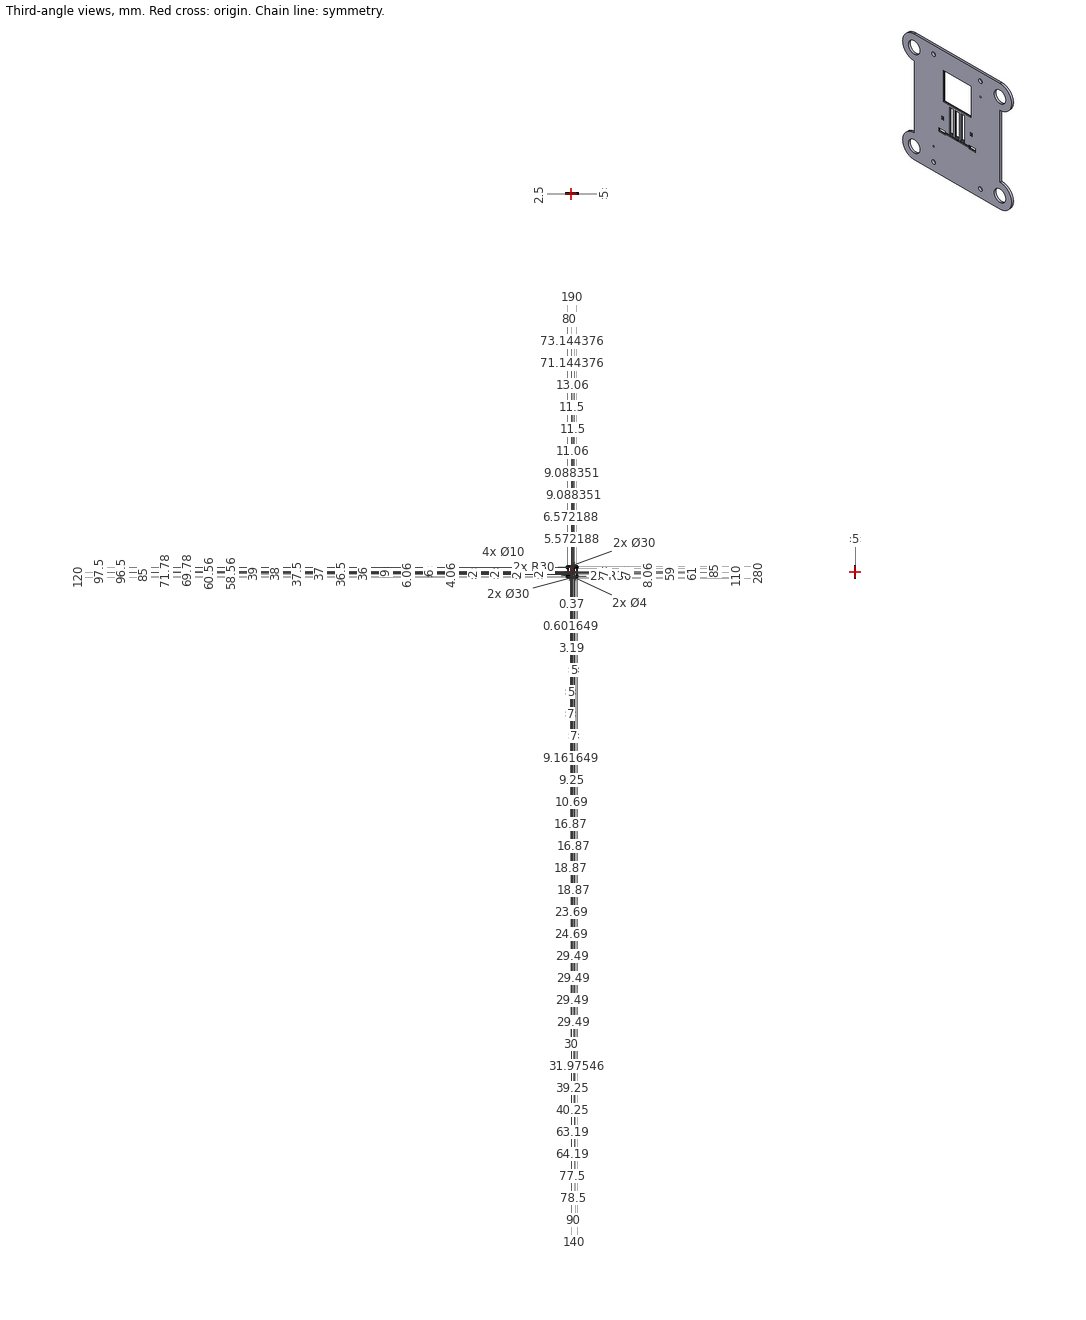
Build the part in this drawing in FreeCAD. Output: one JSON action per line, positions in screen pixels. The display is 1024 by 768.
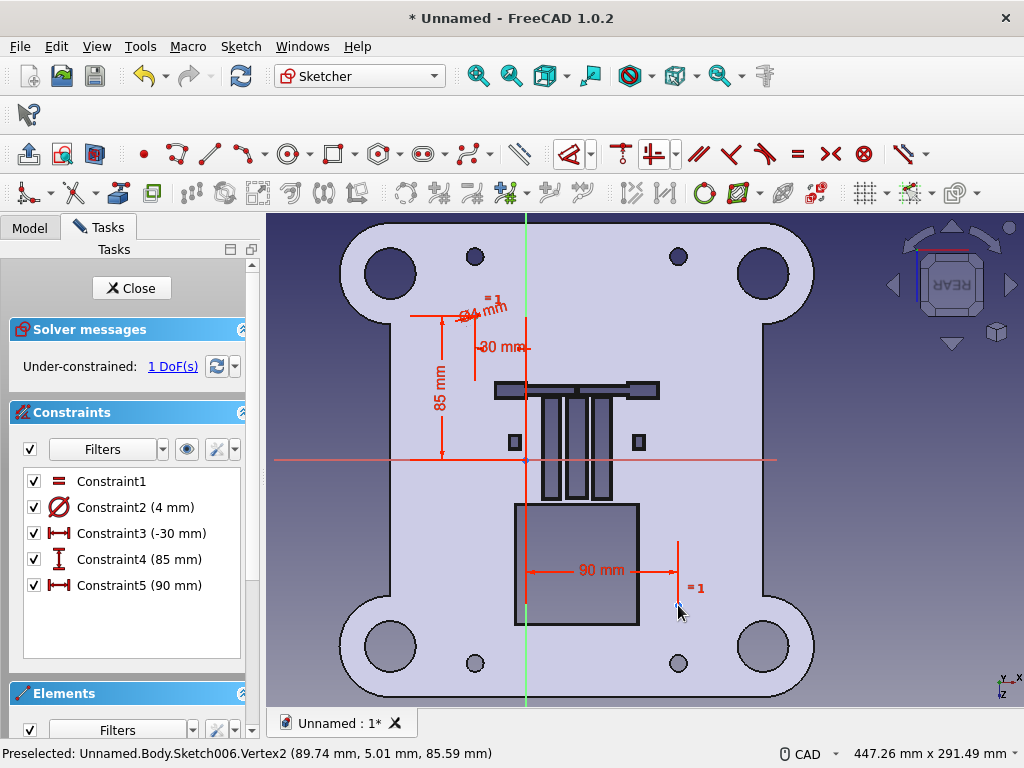
{"action": "left_click", "coordinate": [678, 605]}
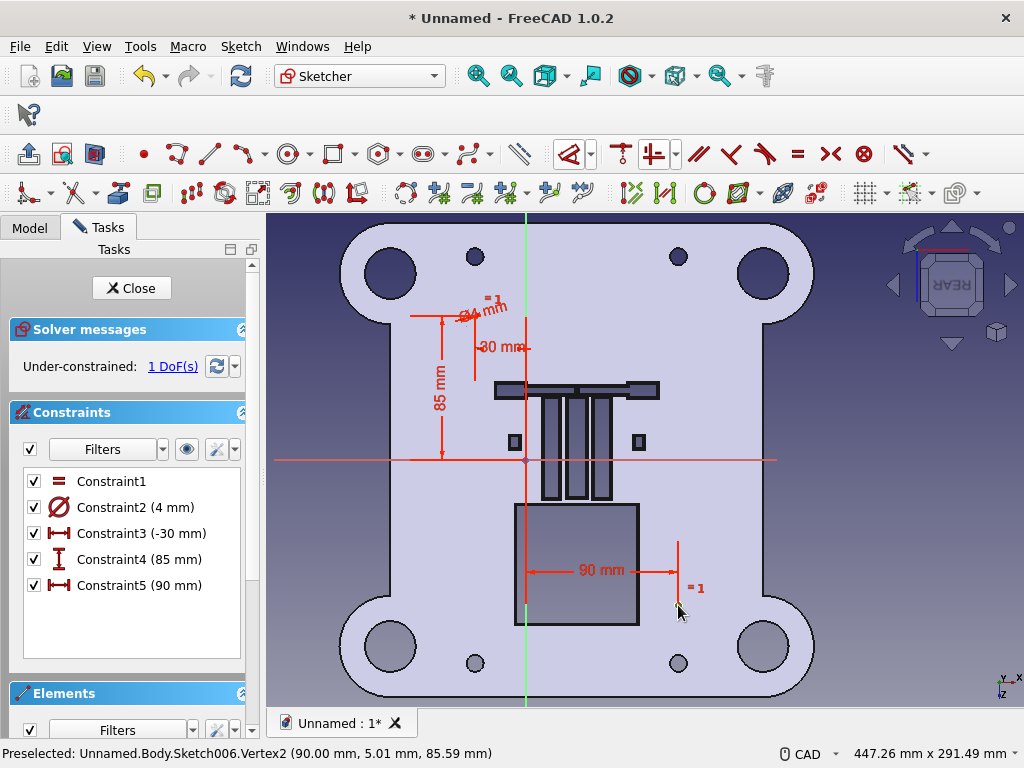
{"action": "left_click", "coordinate": [590, 154]}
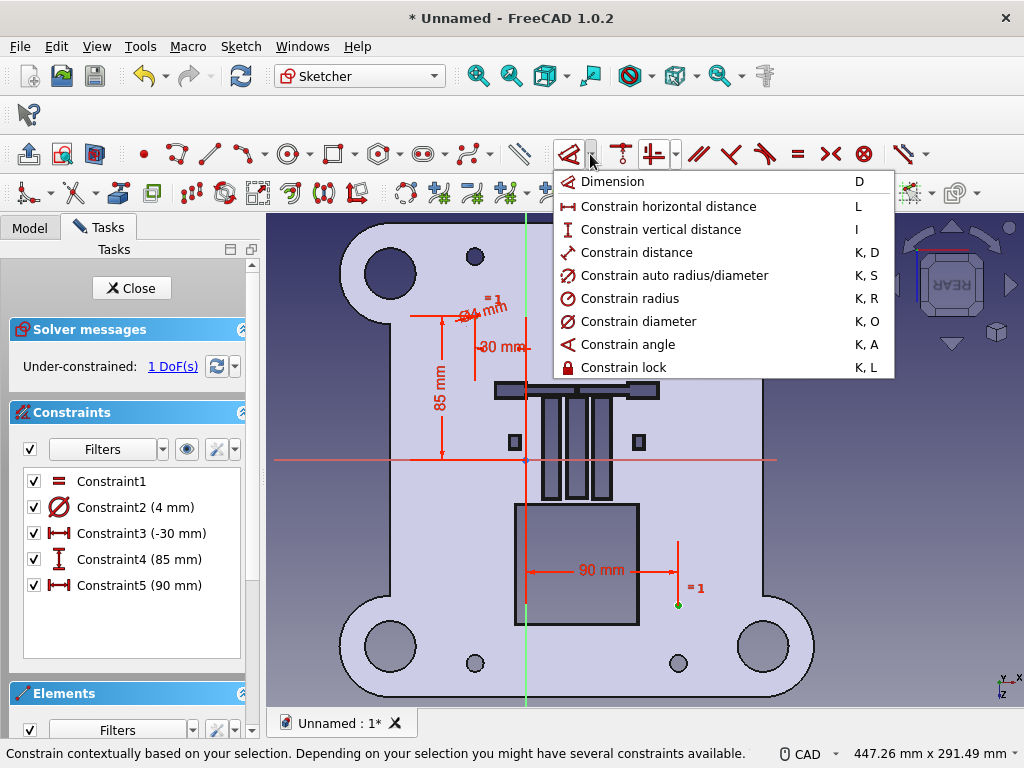
{"action": "left_click", "coordinate": [724, 230]}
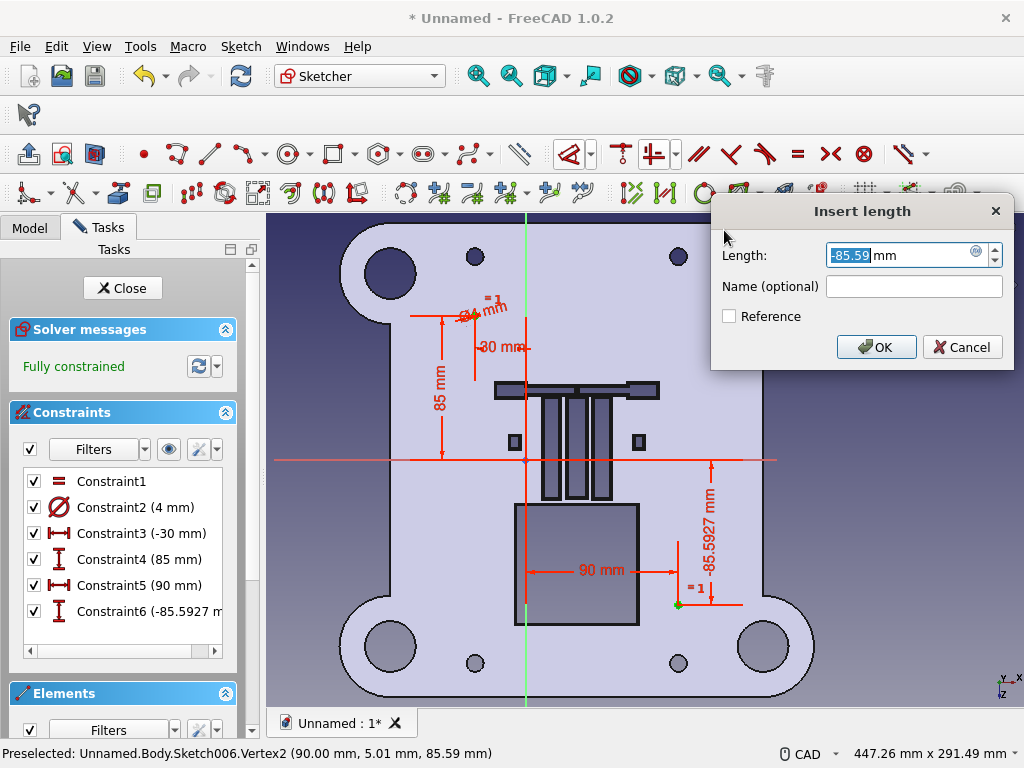
{"action": "type", "text": "-85"}
{"action": "key", "text": "Return"}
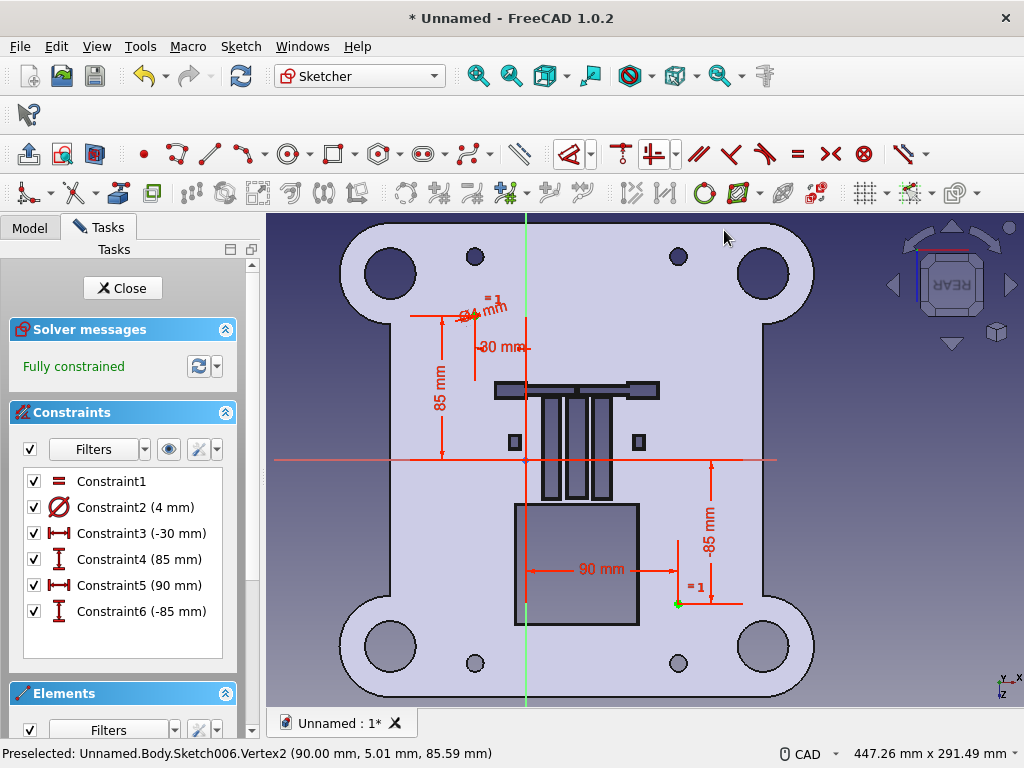
{"action": "left_click", "coordinate": [123, 288]}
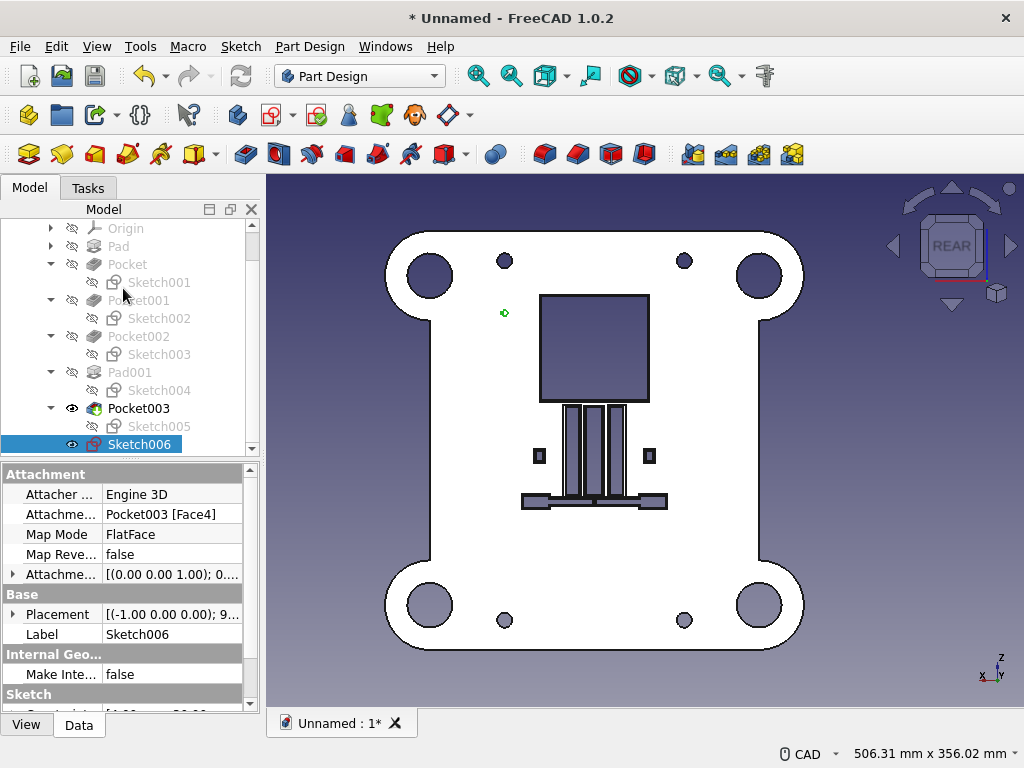
{"action": "left_click", "coordinate": [246, 154]}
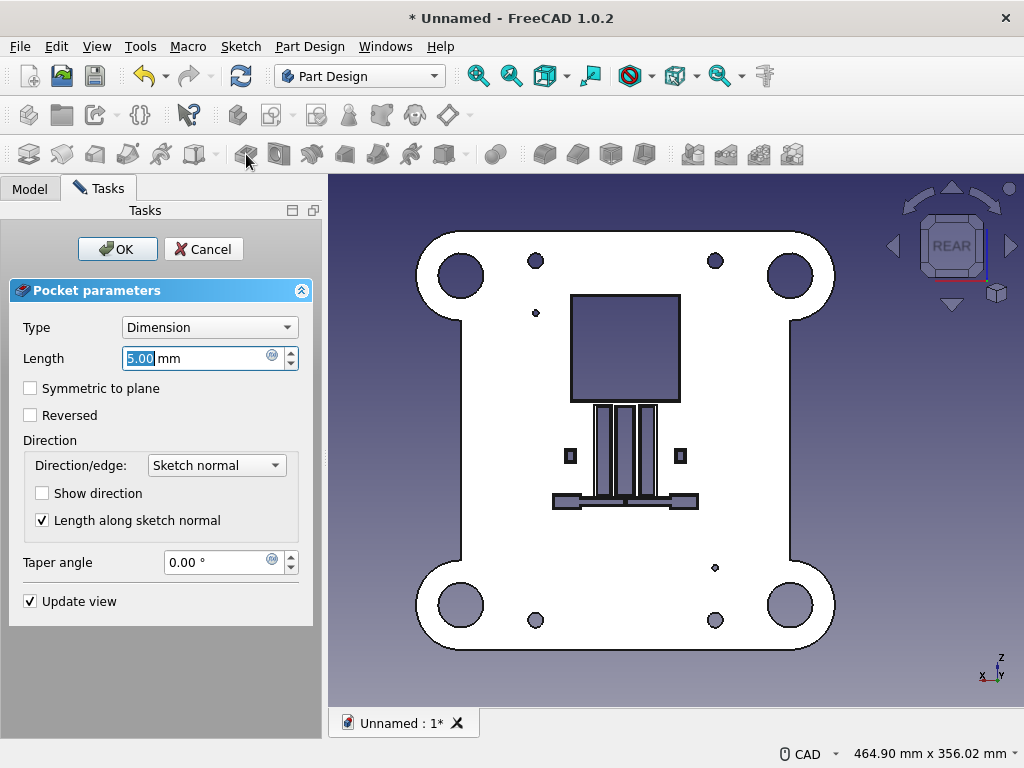
{"action": "left_click", "coordinate": [210, 328]}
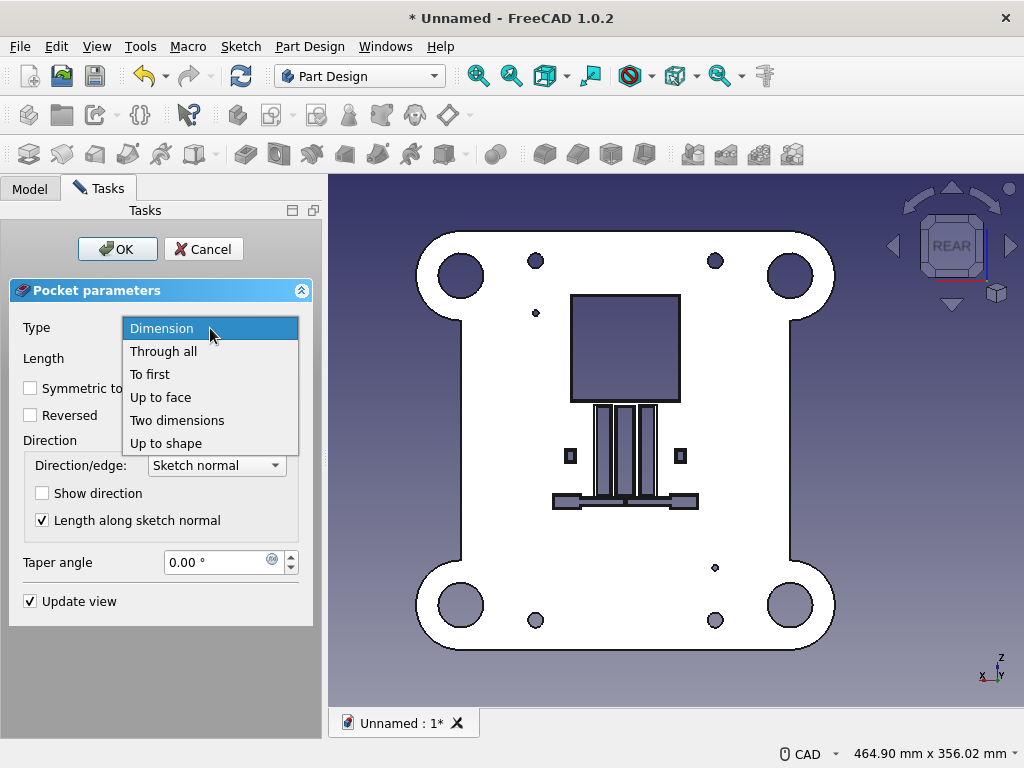
{"action": "left_click", "coordinate": [208, 352]}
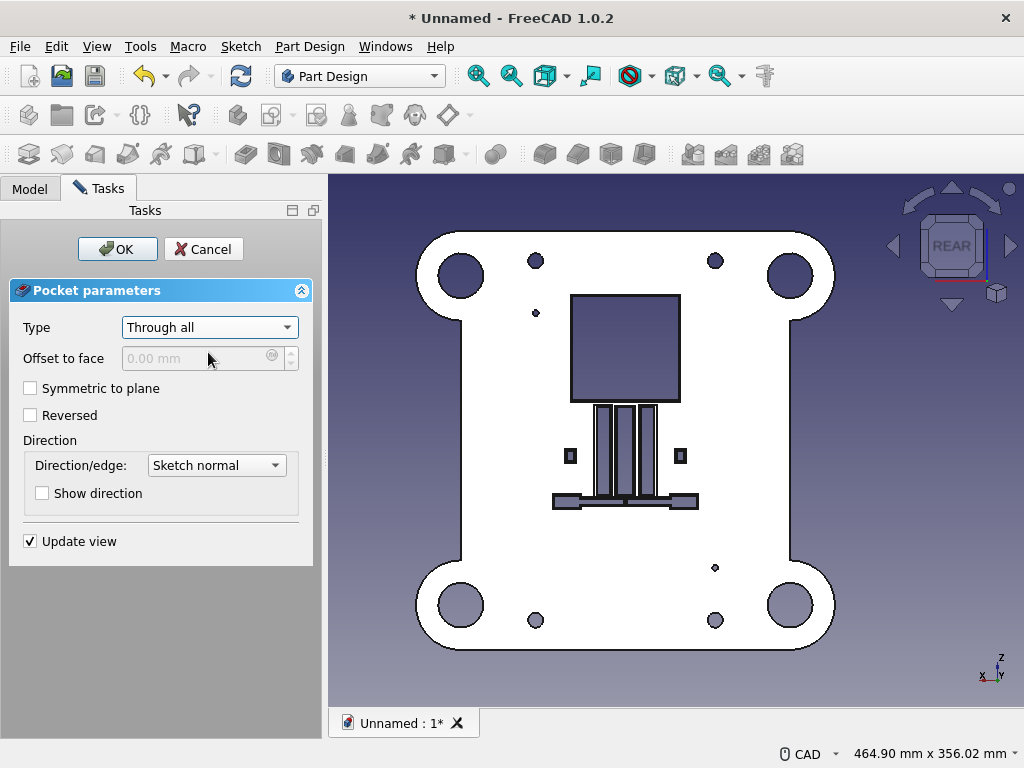
{"action": "left_click", "coordinate": [118, 249]}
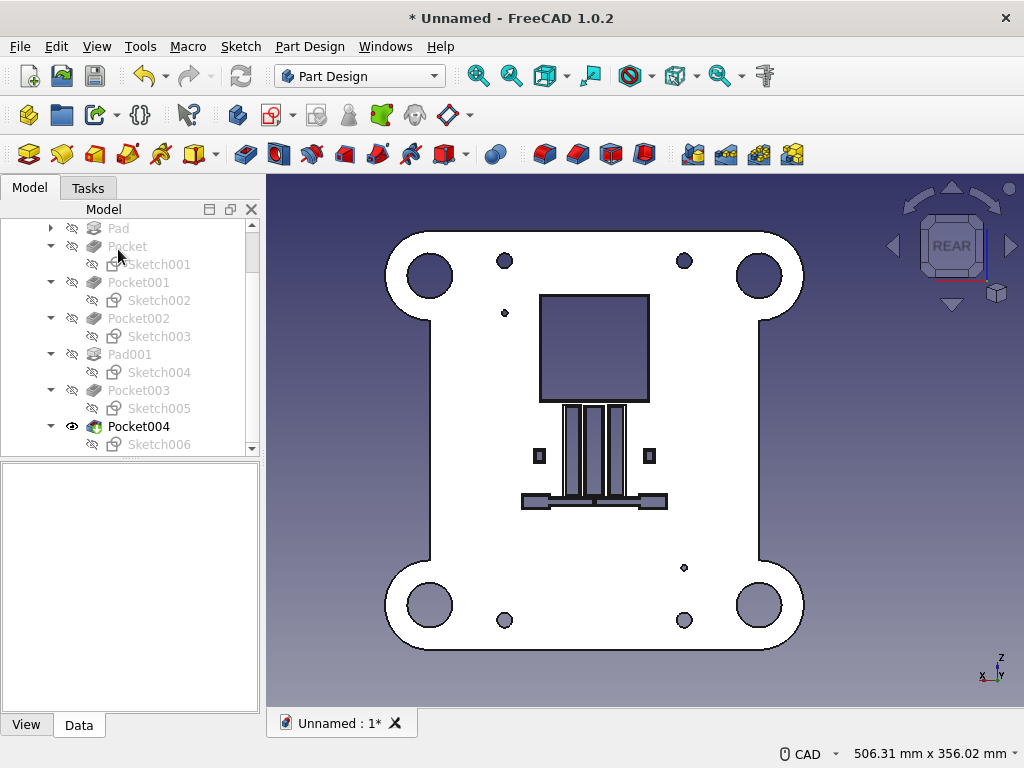
{"action": "key", "text": "0"}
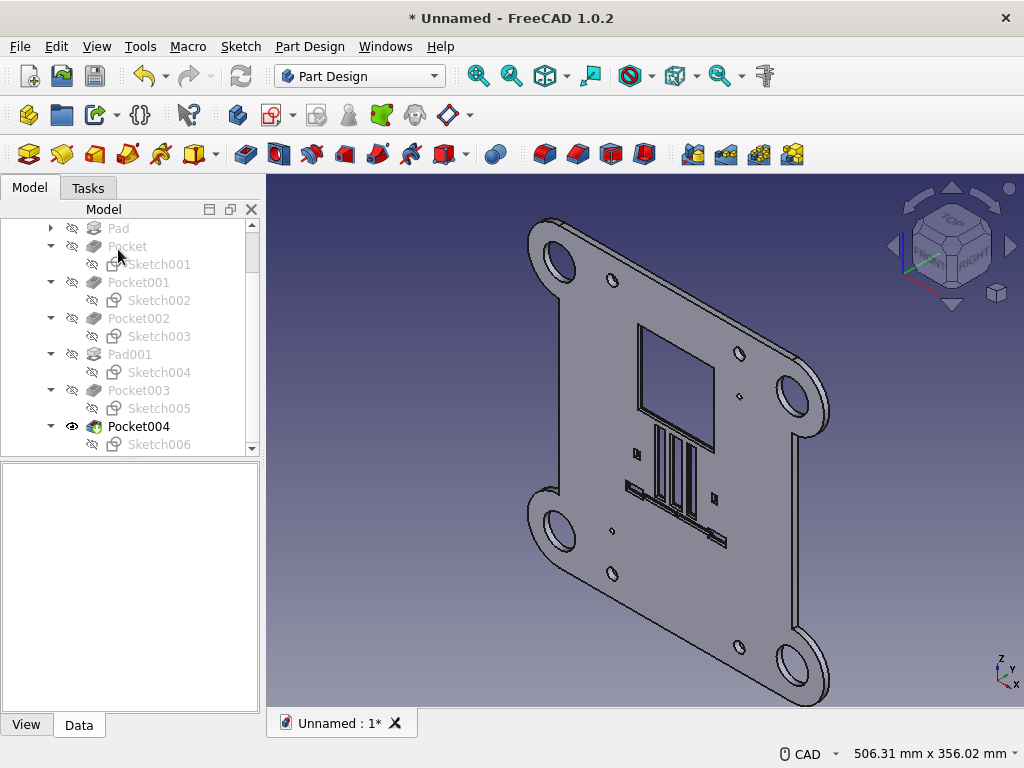
{"action": "left_click", "coordinate": [479, 76]}